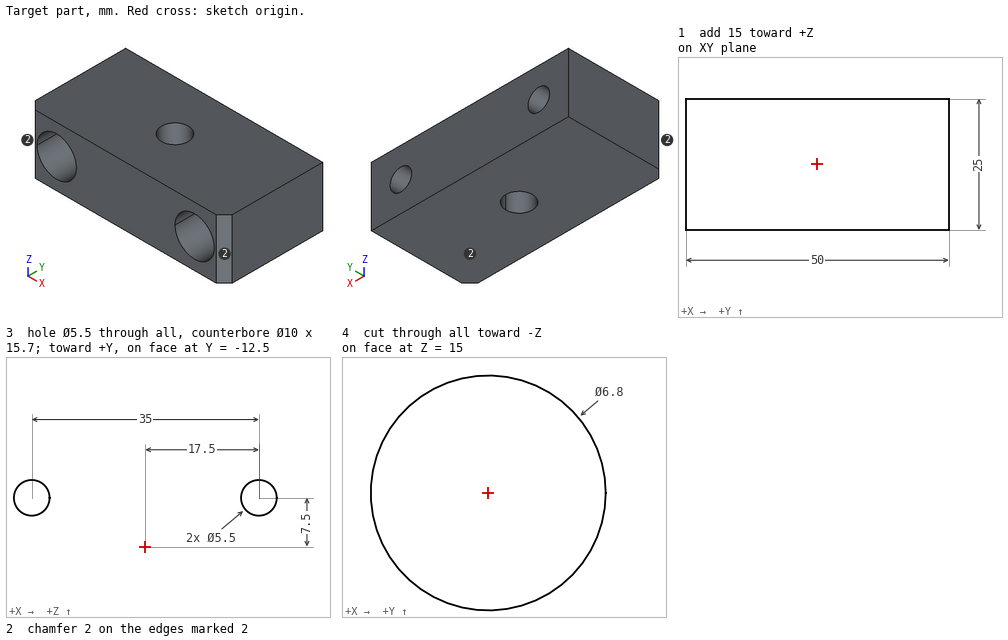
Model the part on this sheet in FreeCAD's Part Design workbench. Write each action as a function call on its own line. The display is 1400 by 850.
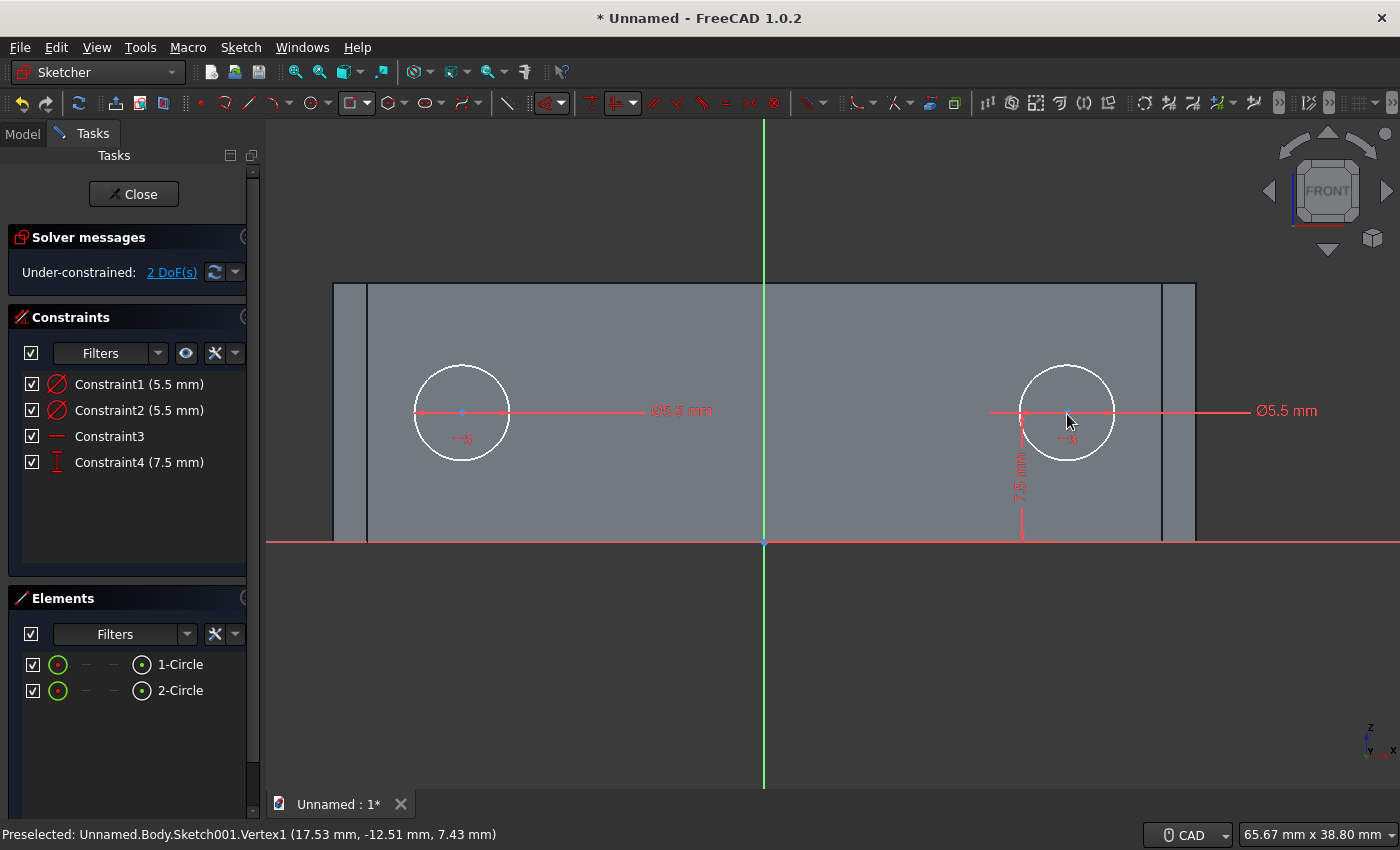
click(1067, 413)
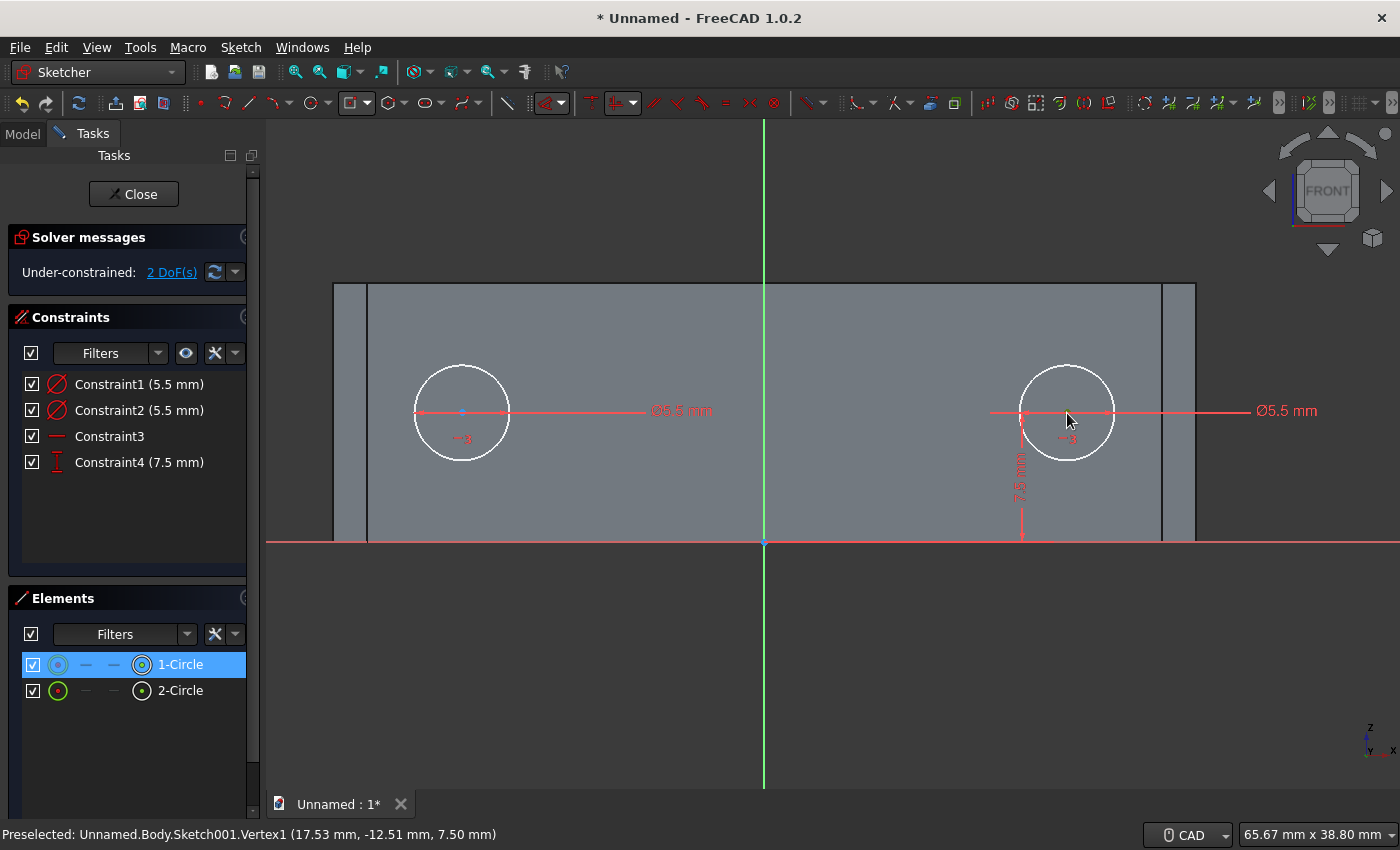
click(462, 413)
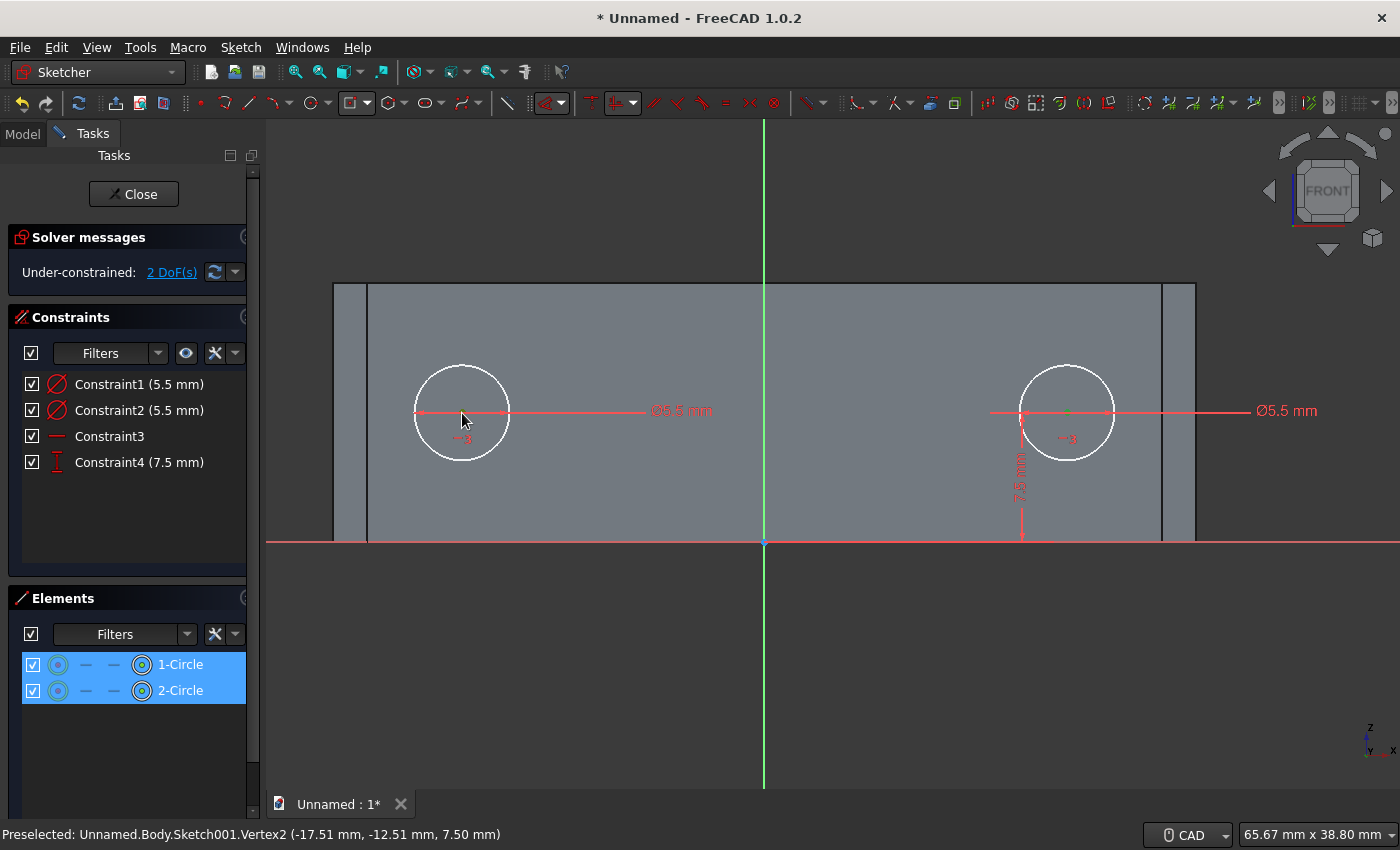
click(564, 104)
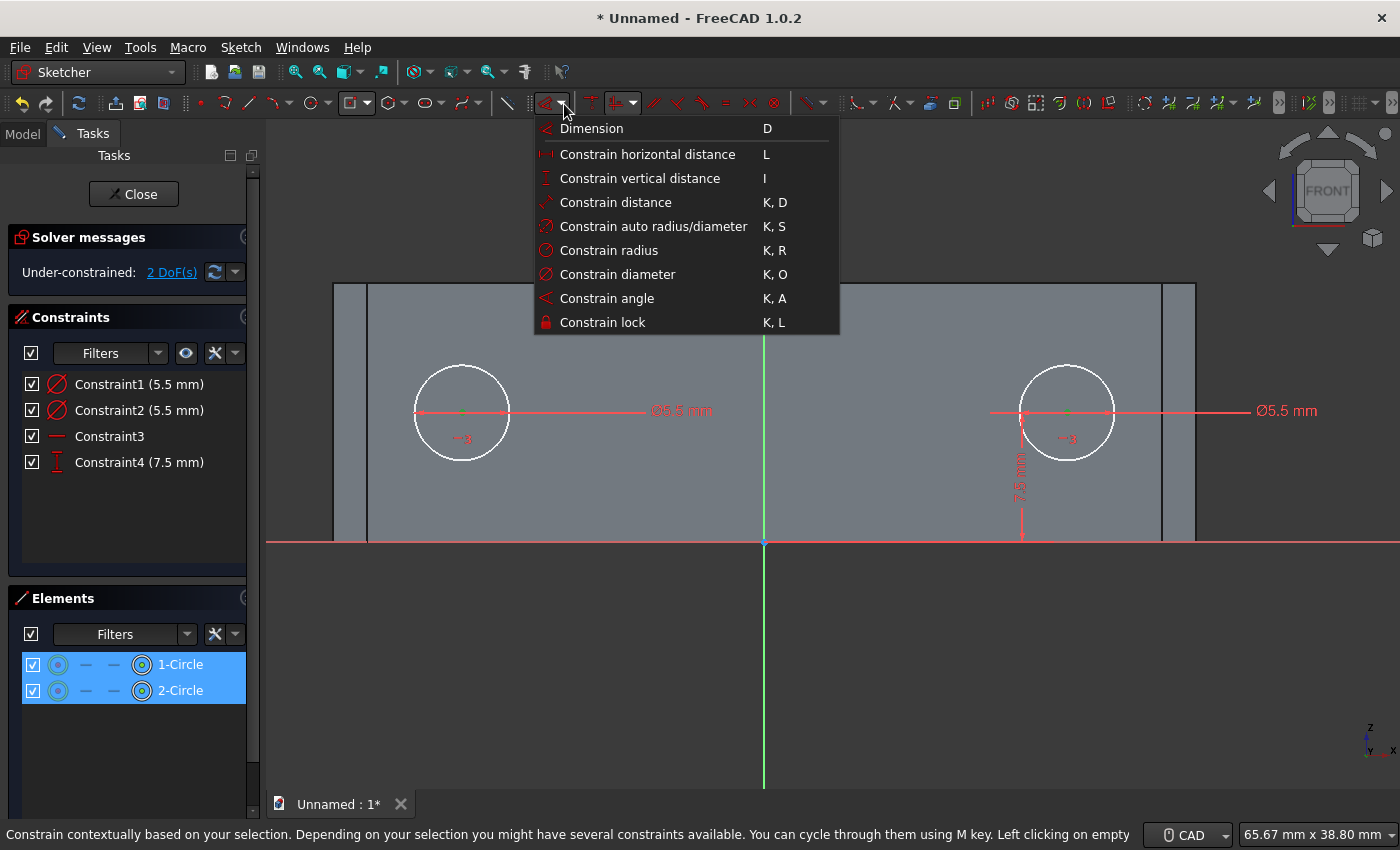
click(687, 154)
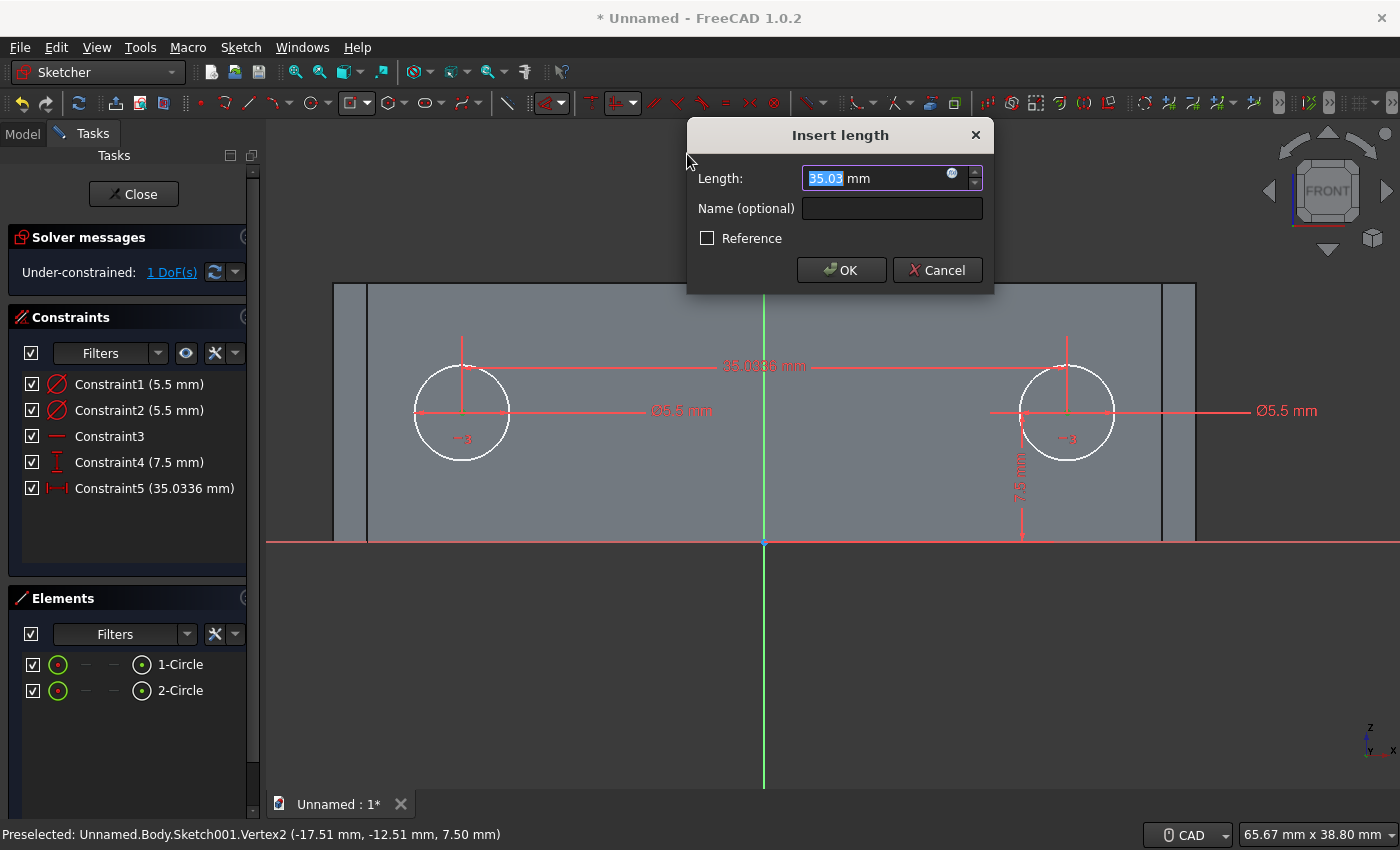
text(35)
key(Return)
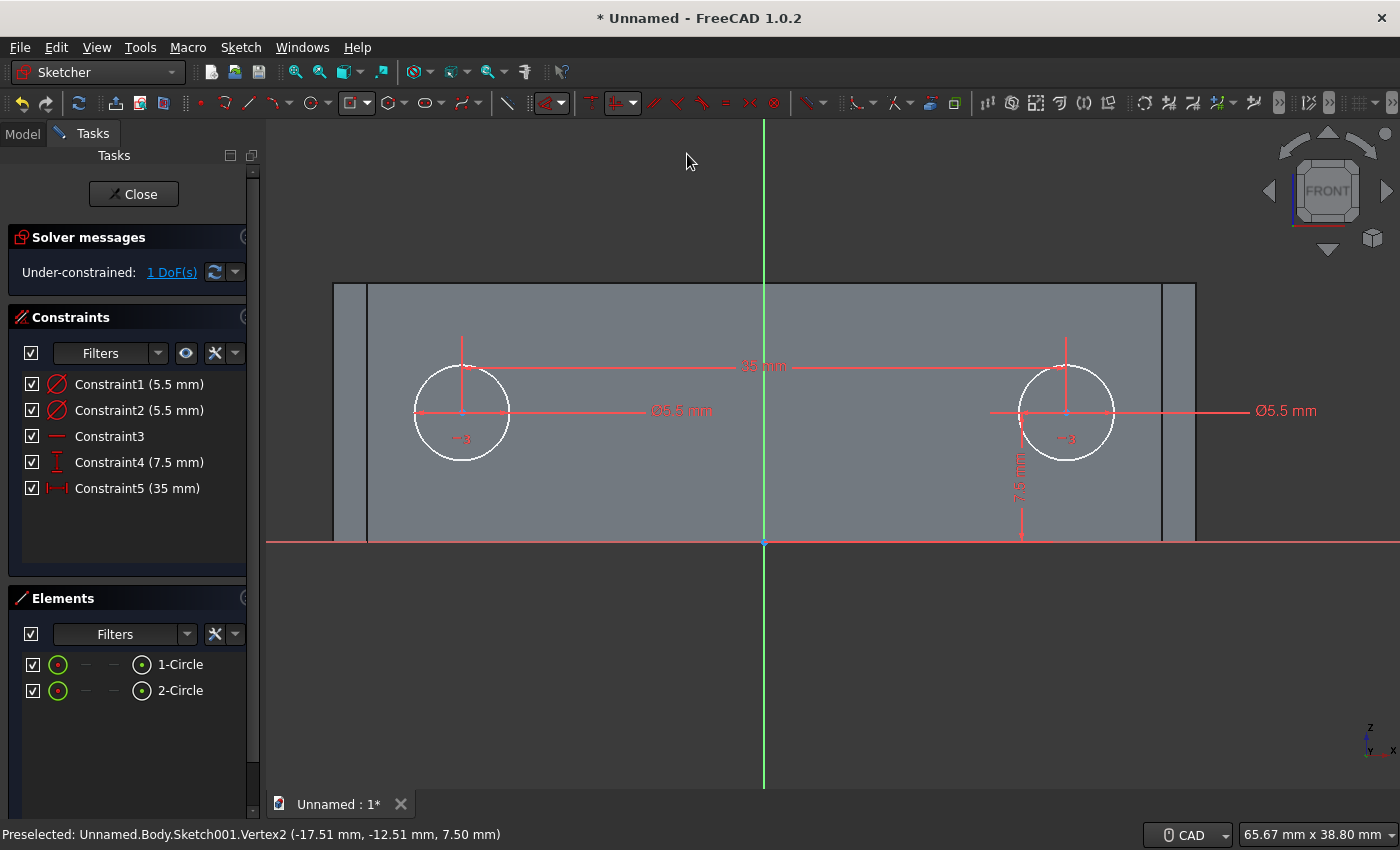
click(1066, 413)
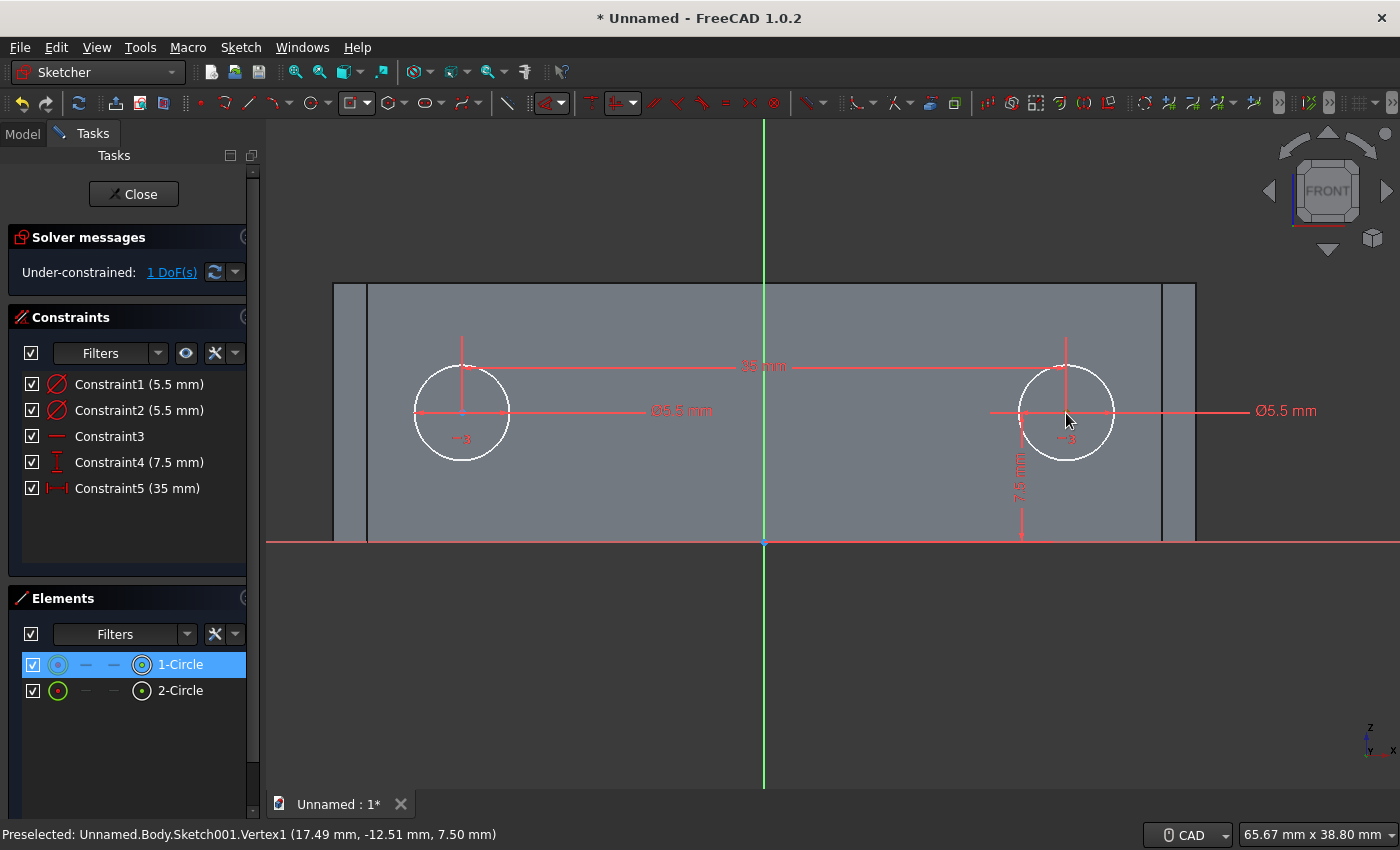
click(564, 104)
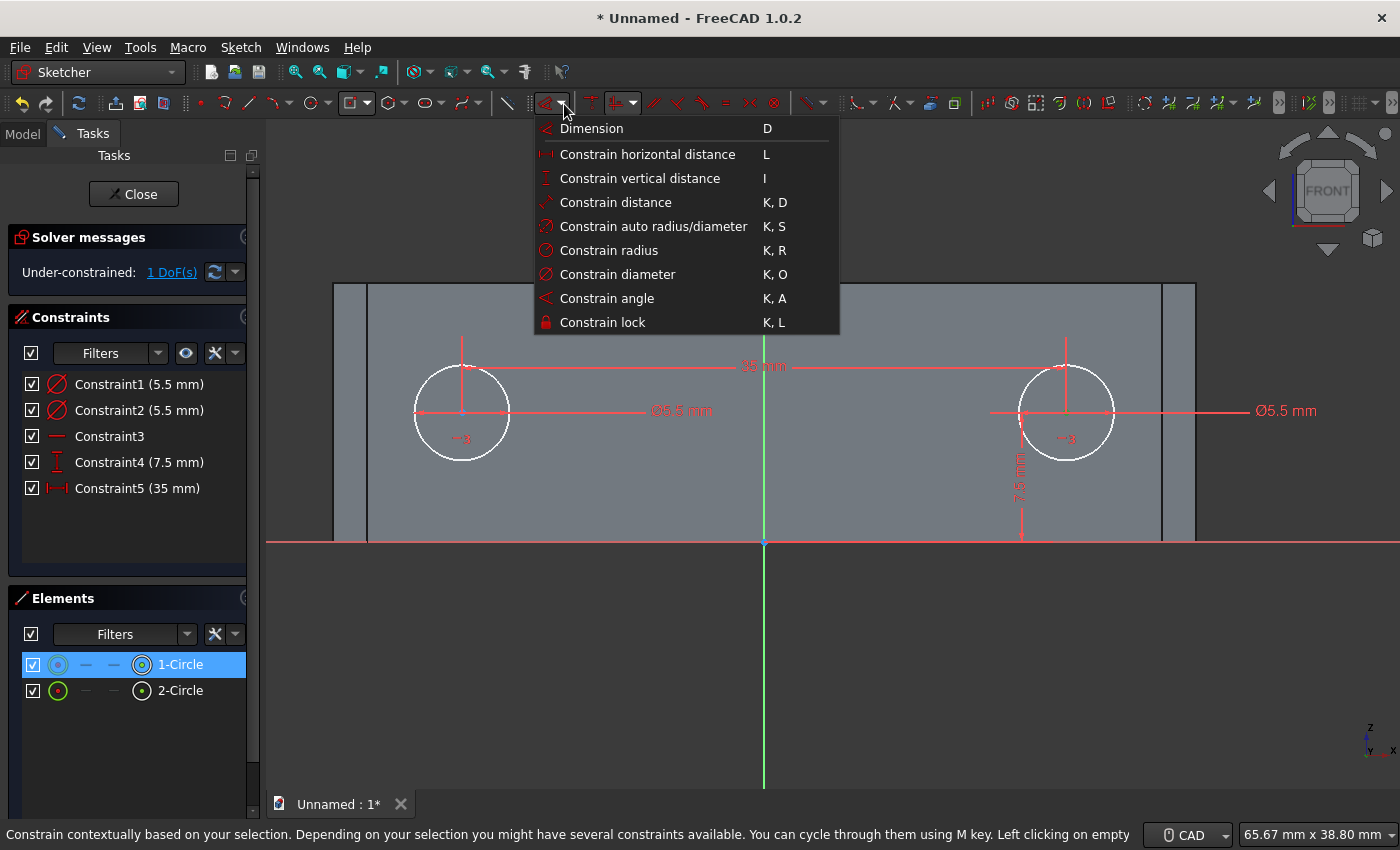
click(687, 154)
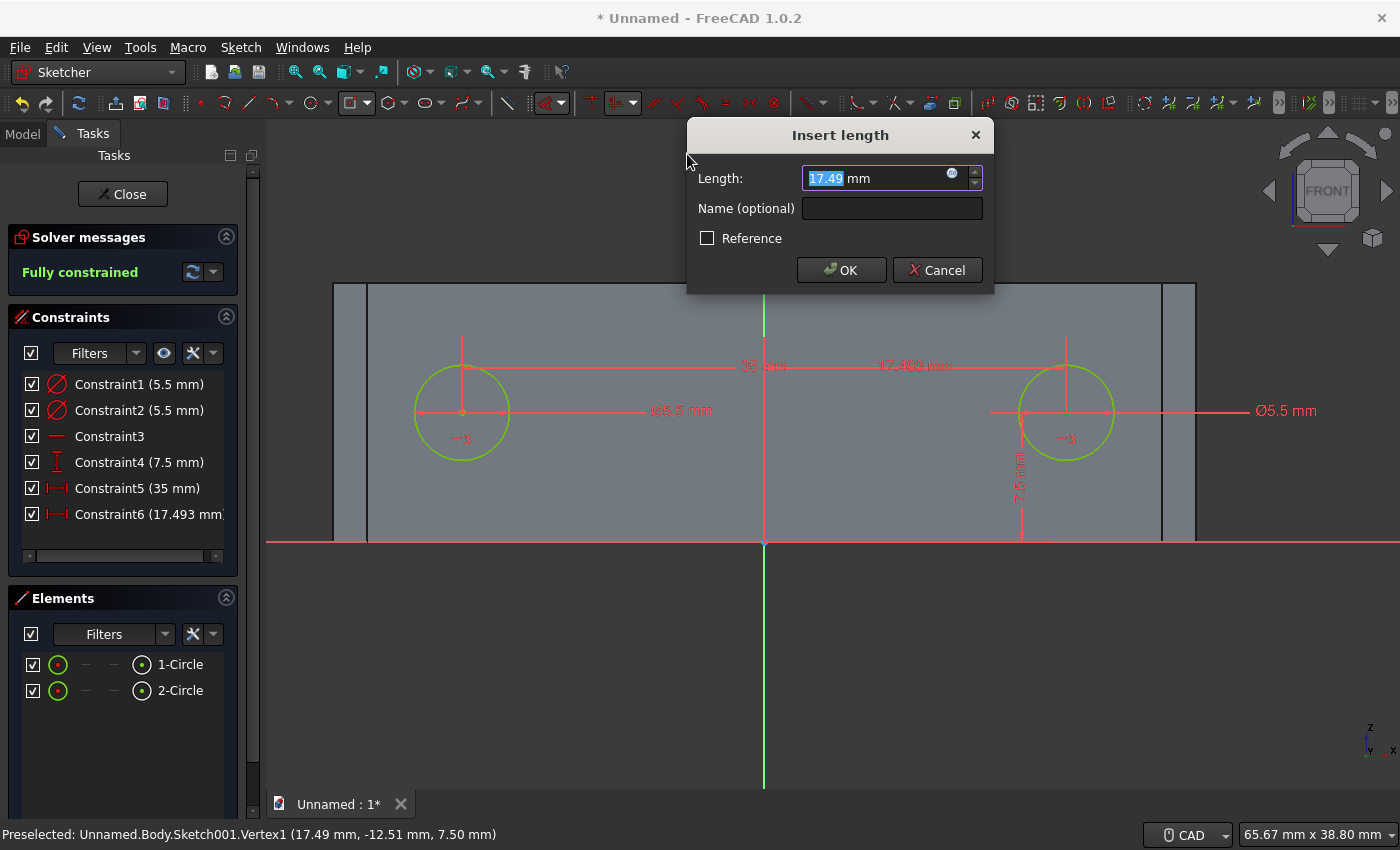
text(17.5)
key(Return)